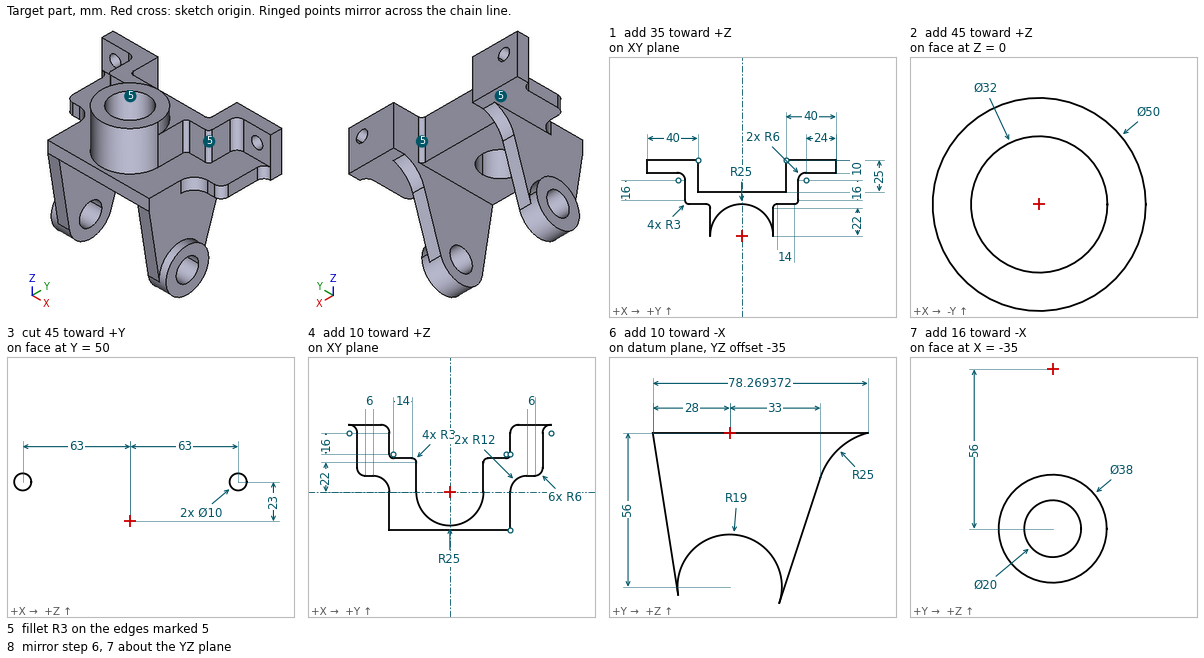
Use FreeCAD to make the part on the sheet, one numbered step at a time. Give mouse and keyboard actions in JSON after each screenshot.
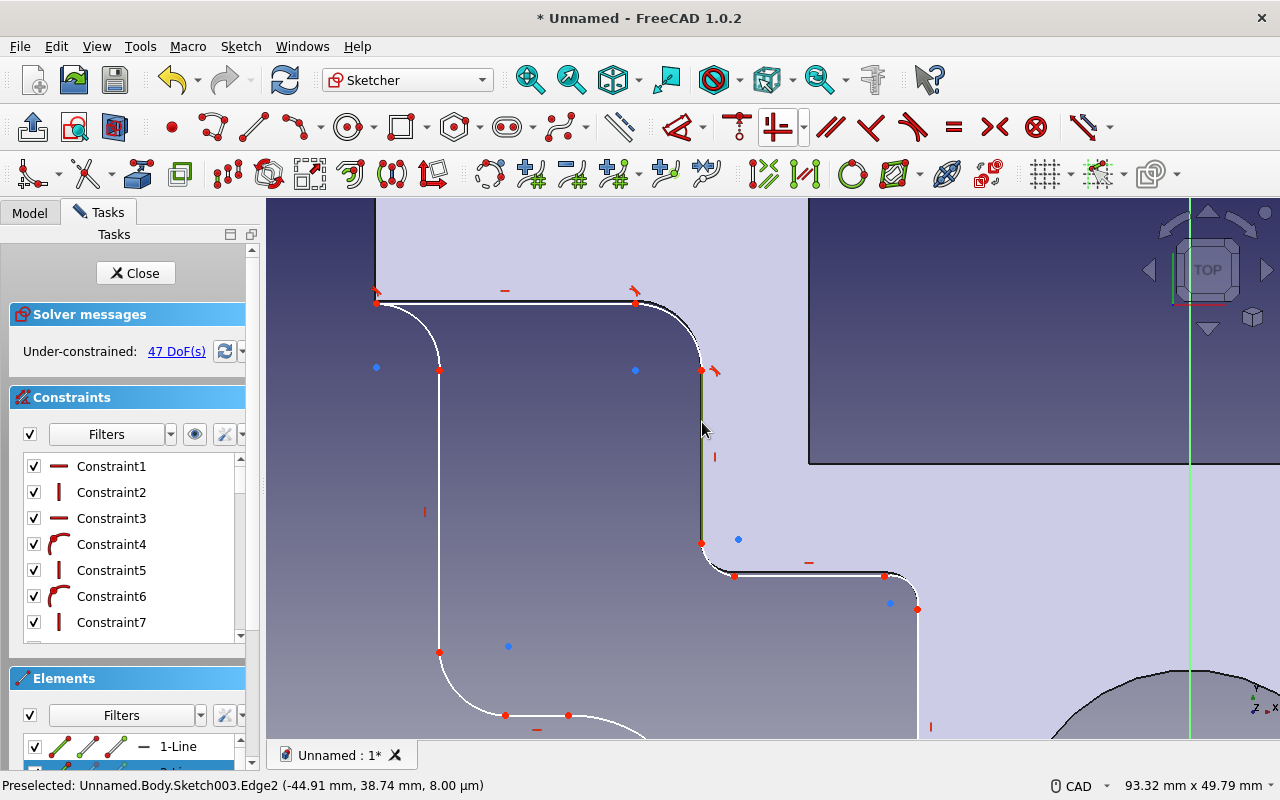
{"action": "left_click", "coordinate": [706, 558]}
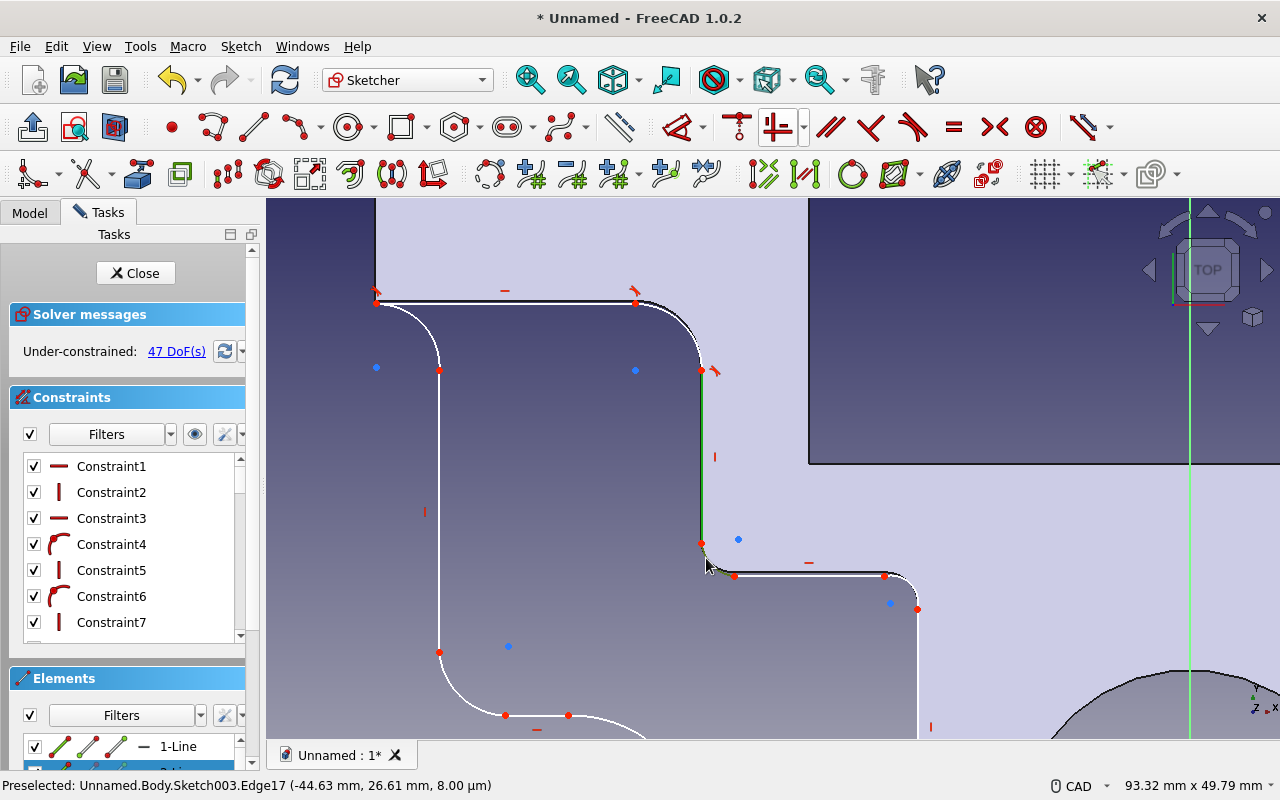
{"action": "left_click", "coordinate": [913, 128]}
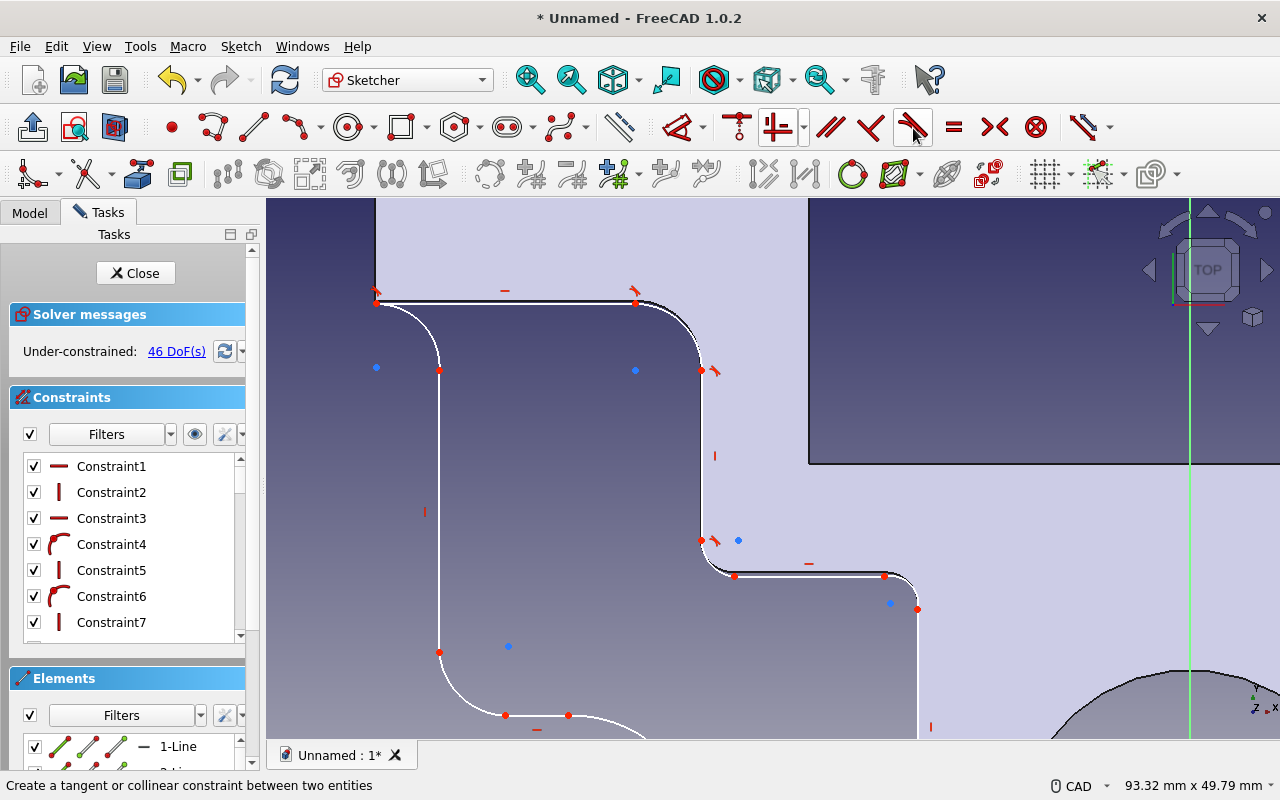
{"action": "left_click", "coordinate": [780, 577]}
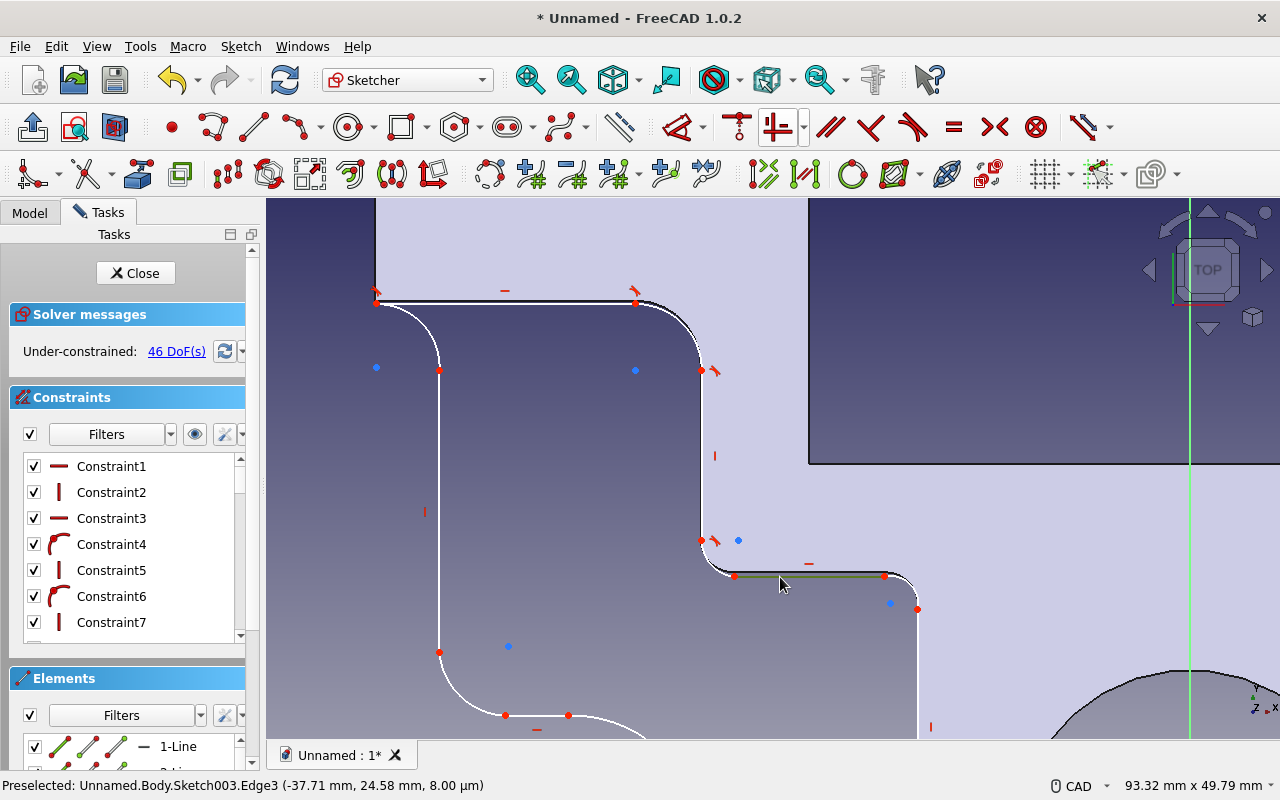
{"action": "left_click", "coordinate": [705, 556]}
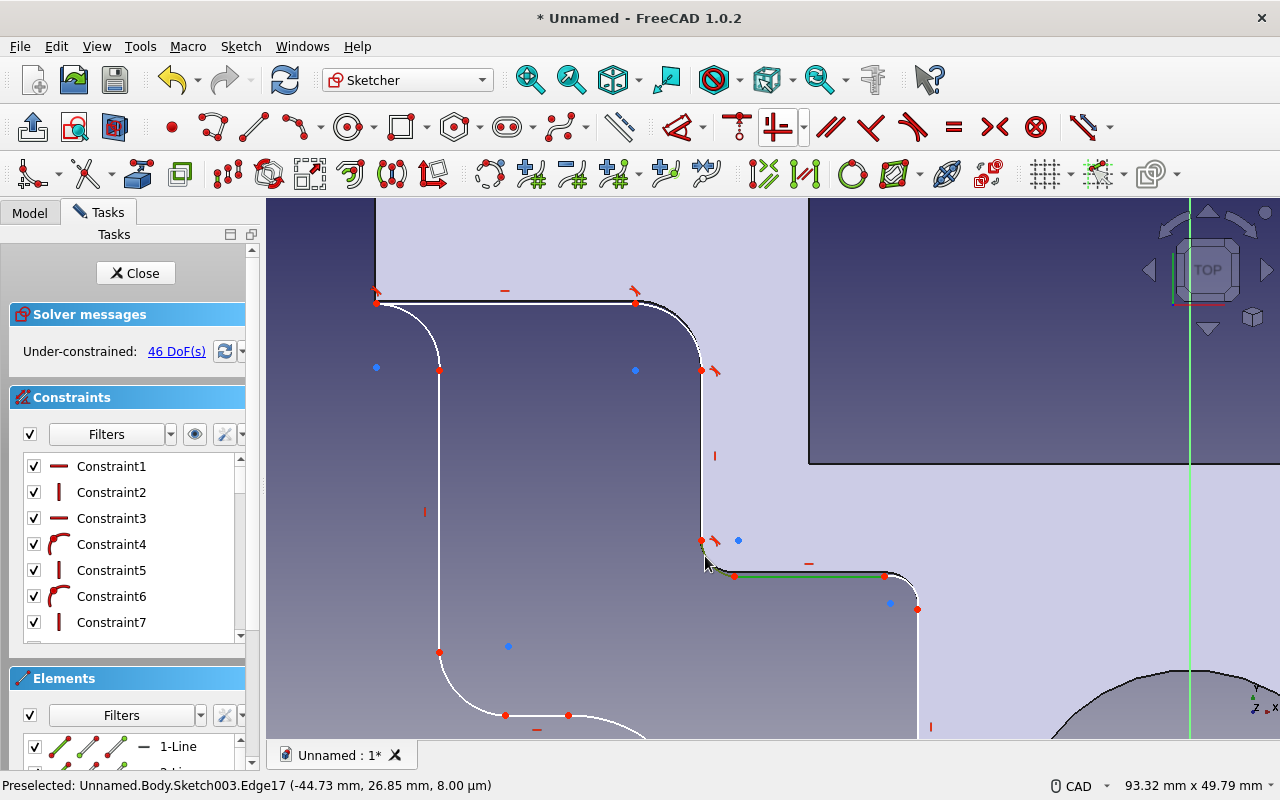
{"action": "left_click", "coordinate": [913, 128]}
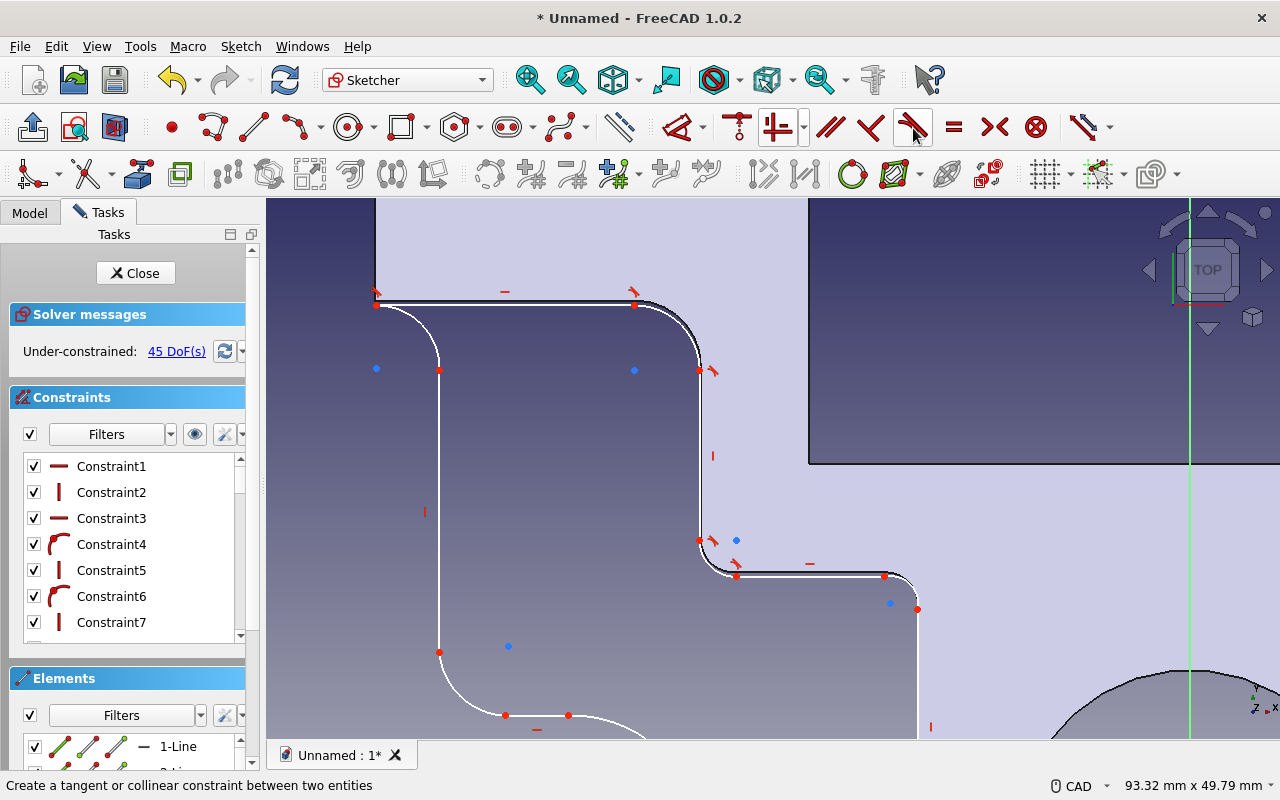
{"action": "left_click", "coordinate": [781, 577]}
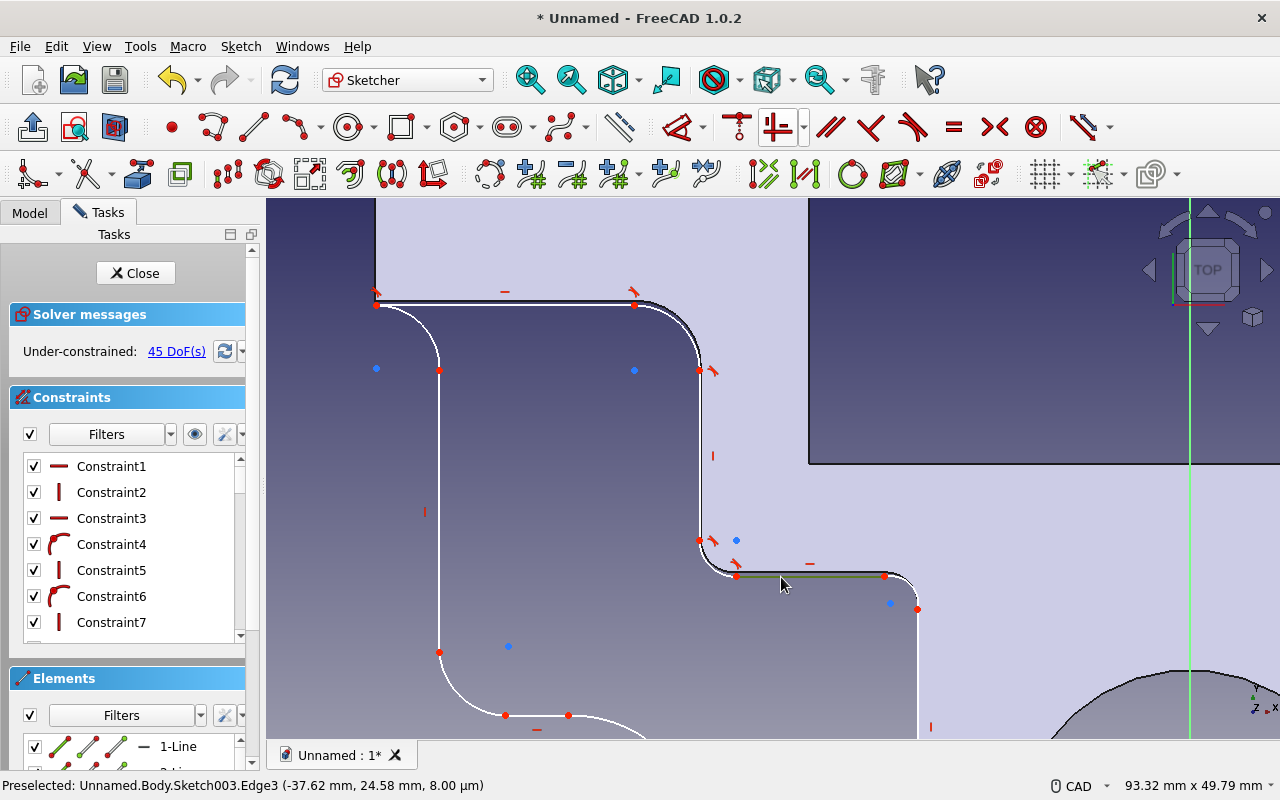
{"action": "left_click", "coordinate": [916, 593]}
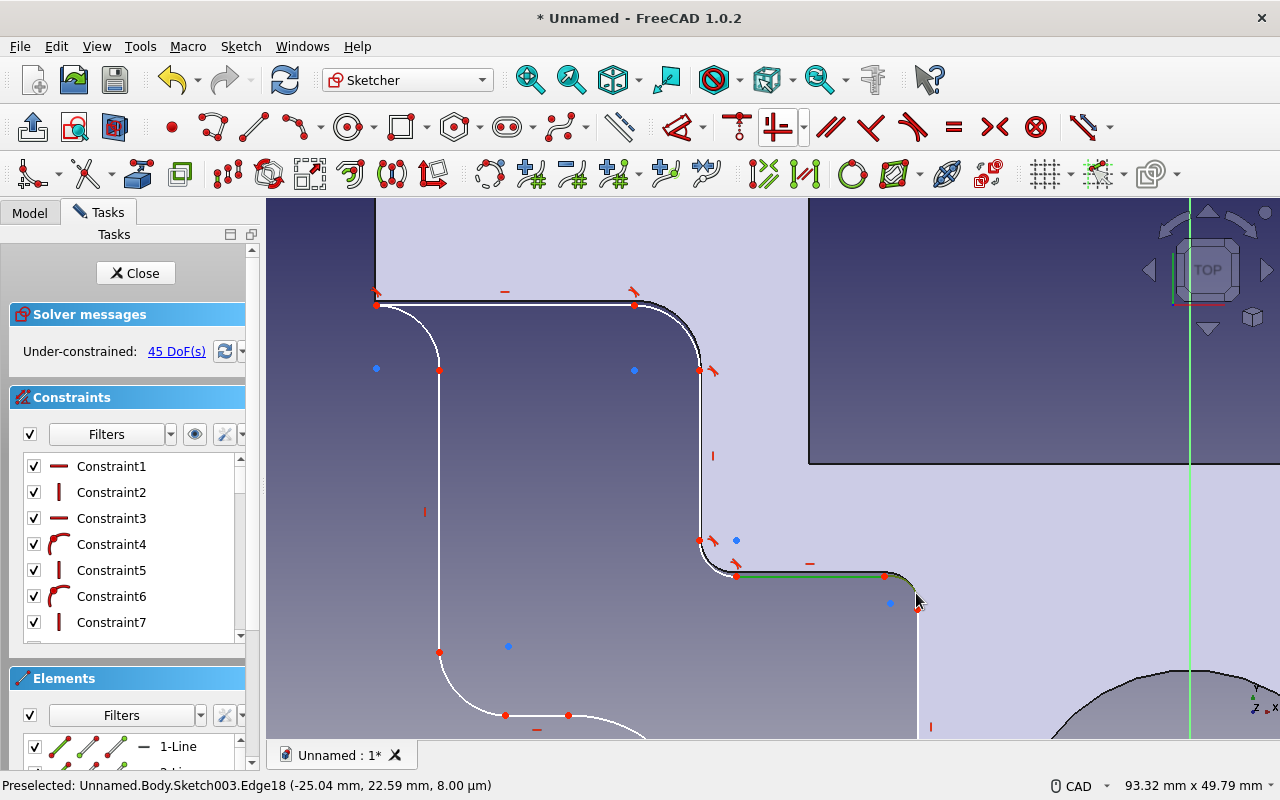
{"action": "left_click", "coordinate": [913, 128]}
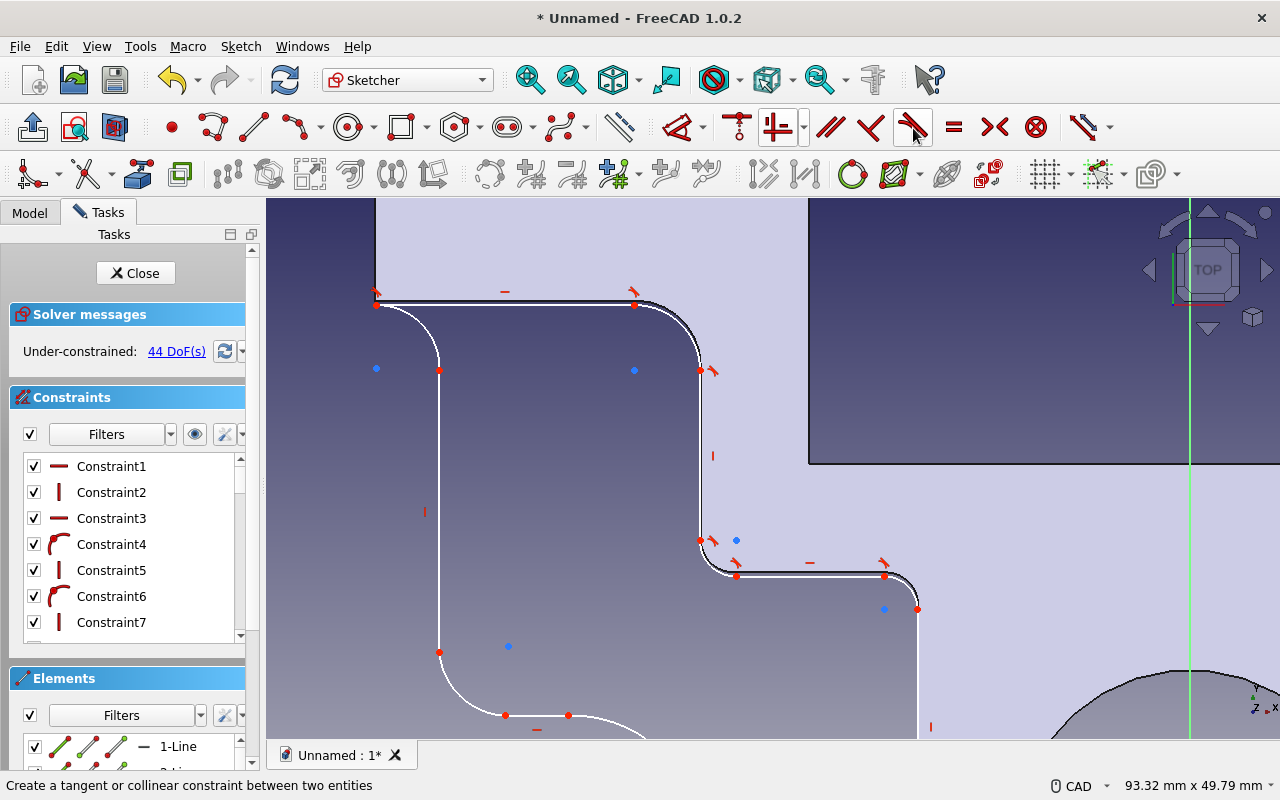
{"action": "left_click", "coordinate": [918, 680]}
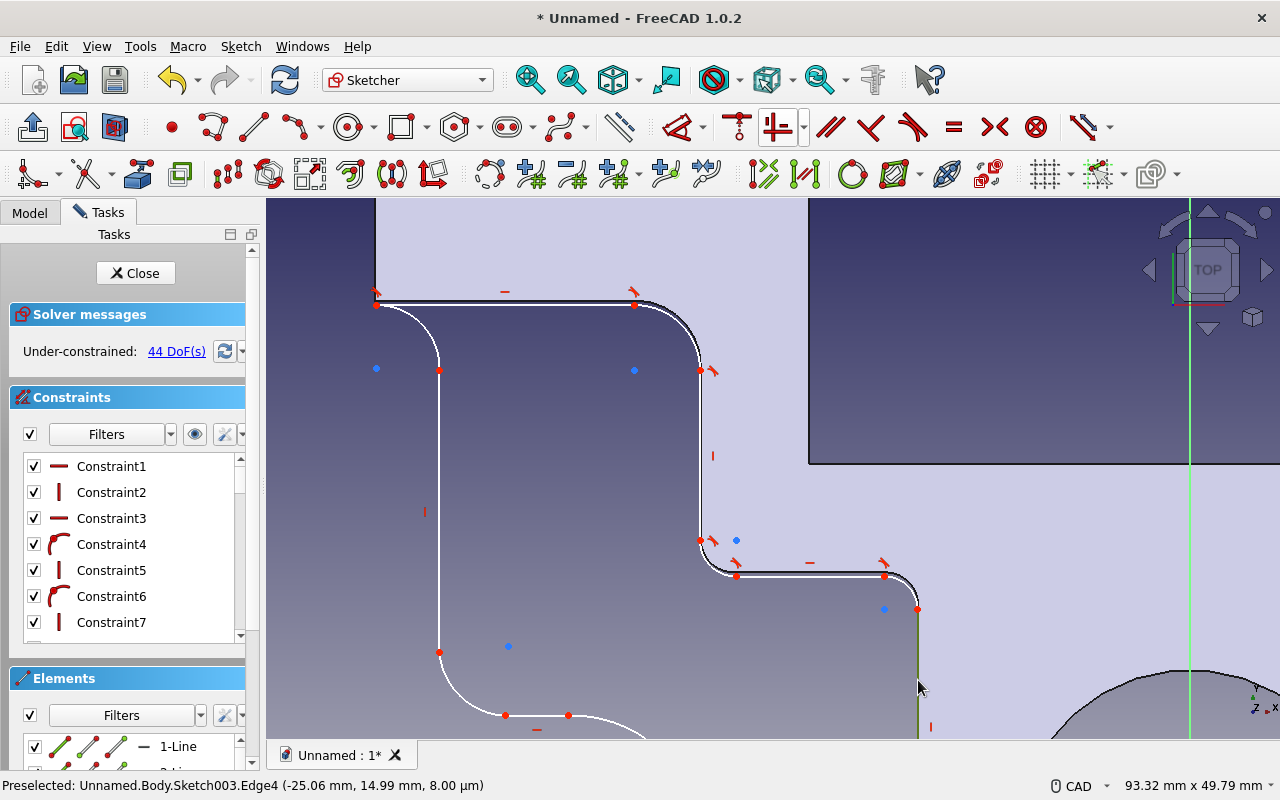
{"action": "left_click", "coordinate": [914, 594]}